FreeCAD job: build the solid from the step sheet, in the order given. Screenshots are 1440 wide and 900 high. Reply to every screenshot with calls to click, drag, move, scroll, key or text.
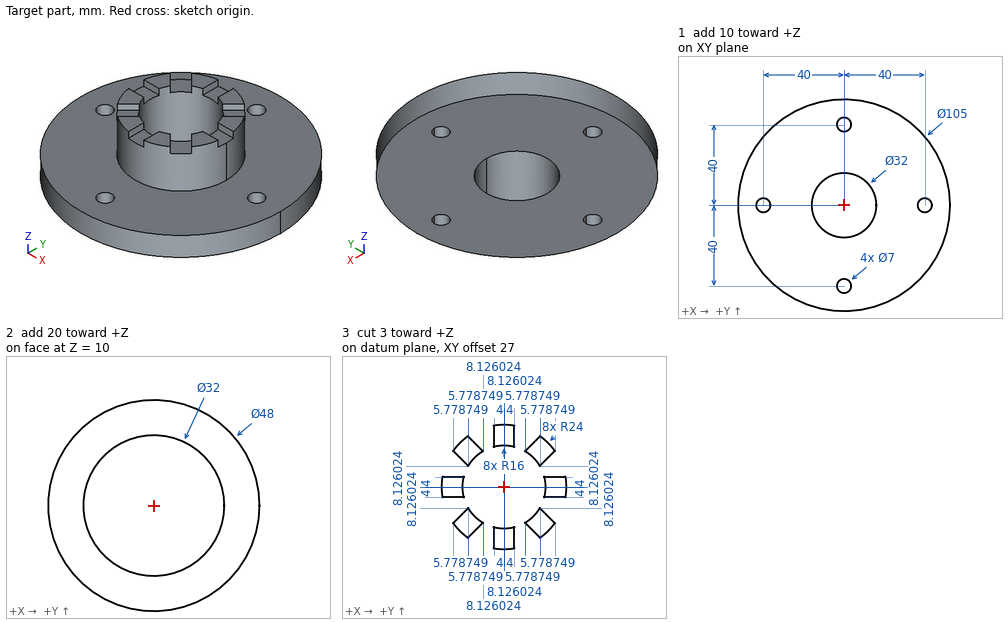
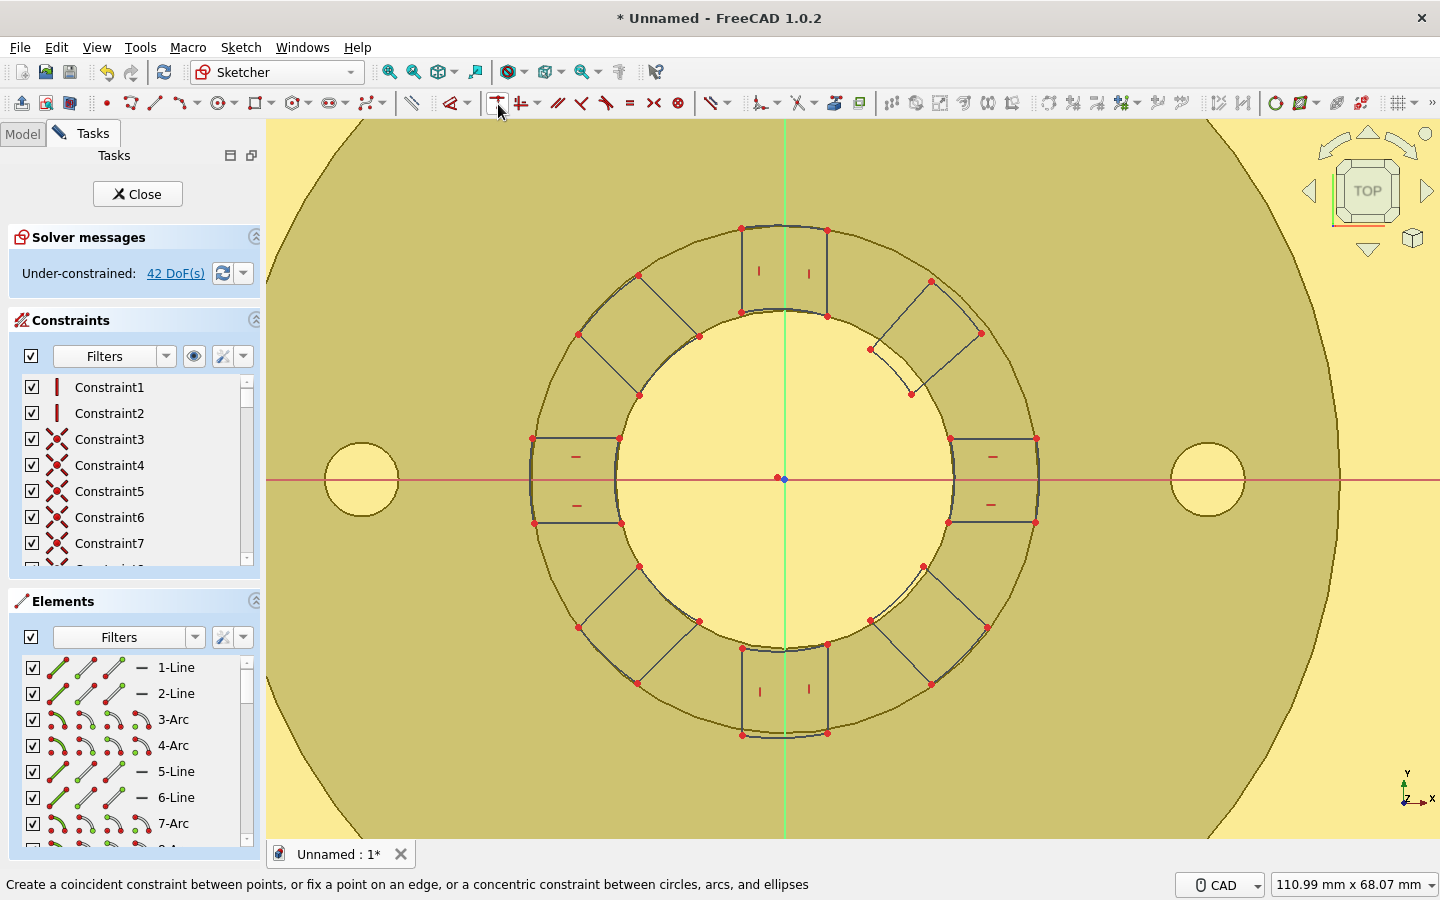
drag(768, 467, 795, 490)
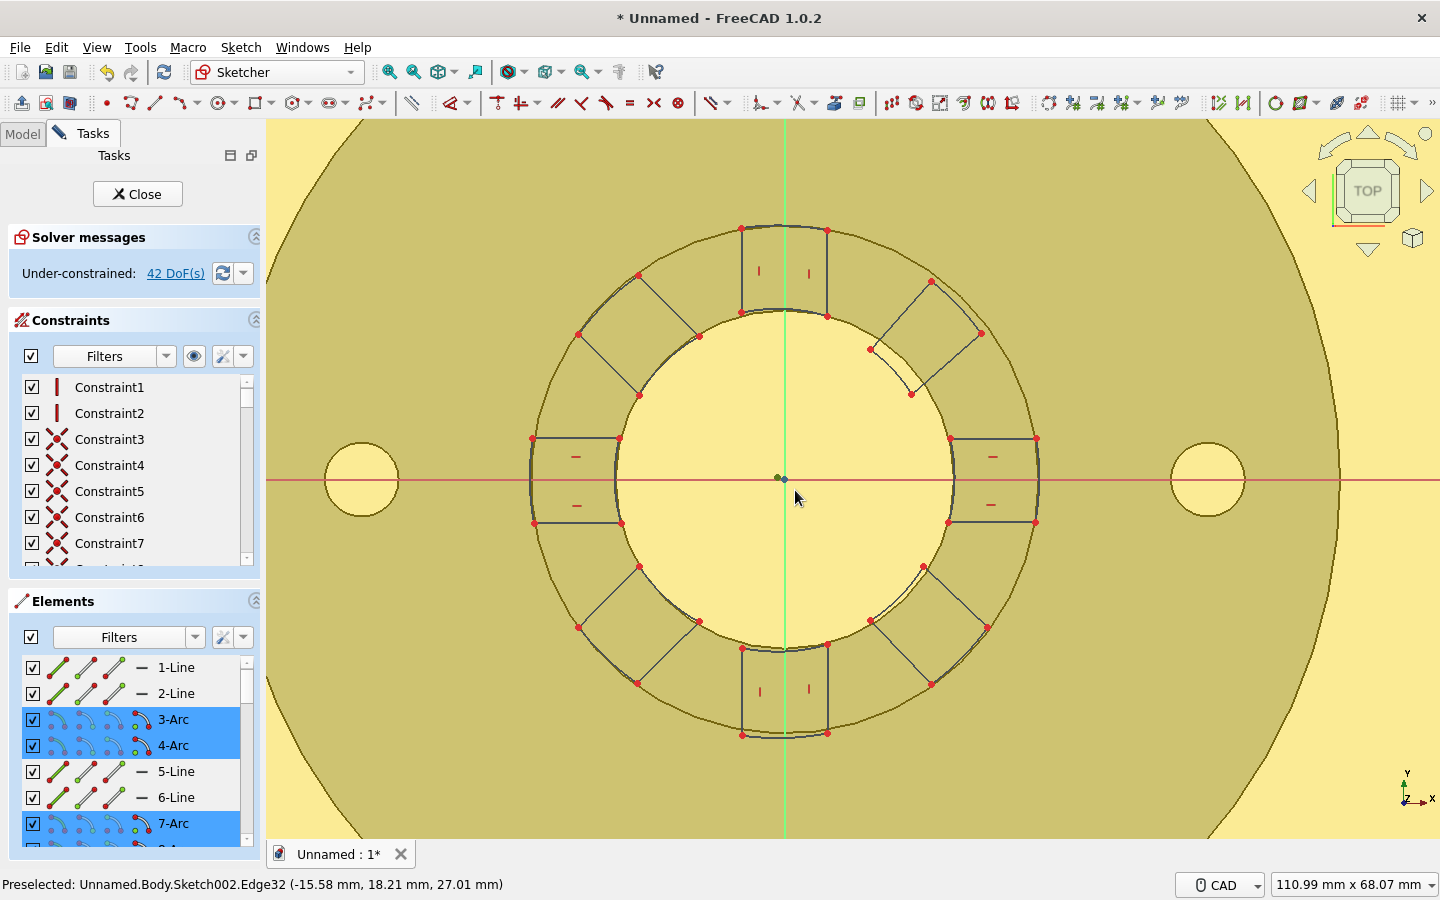
click(498, 104)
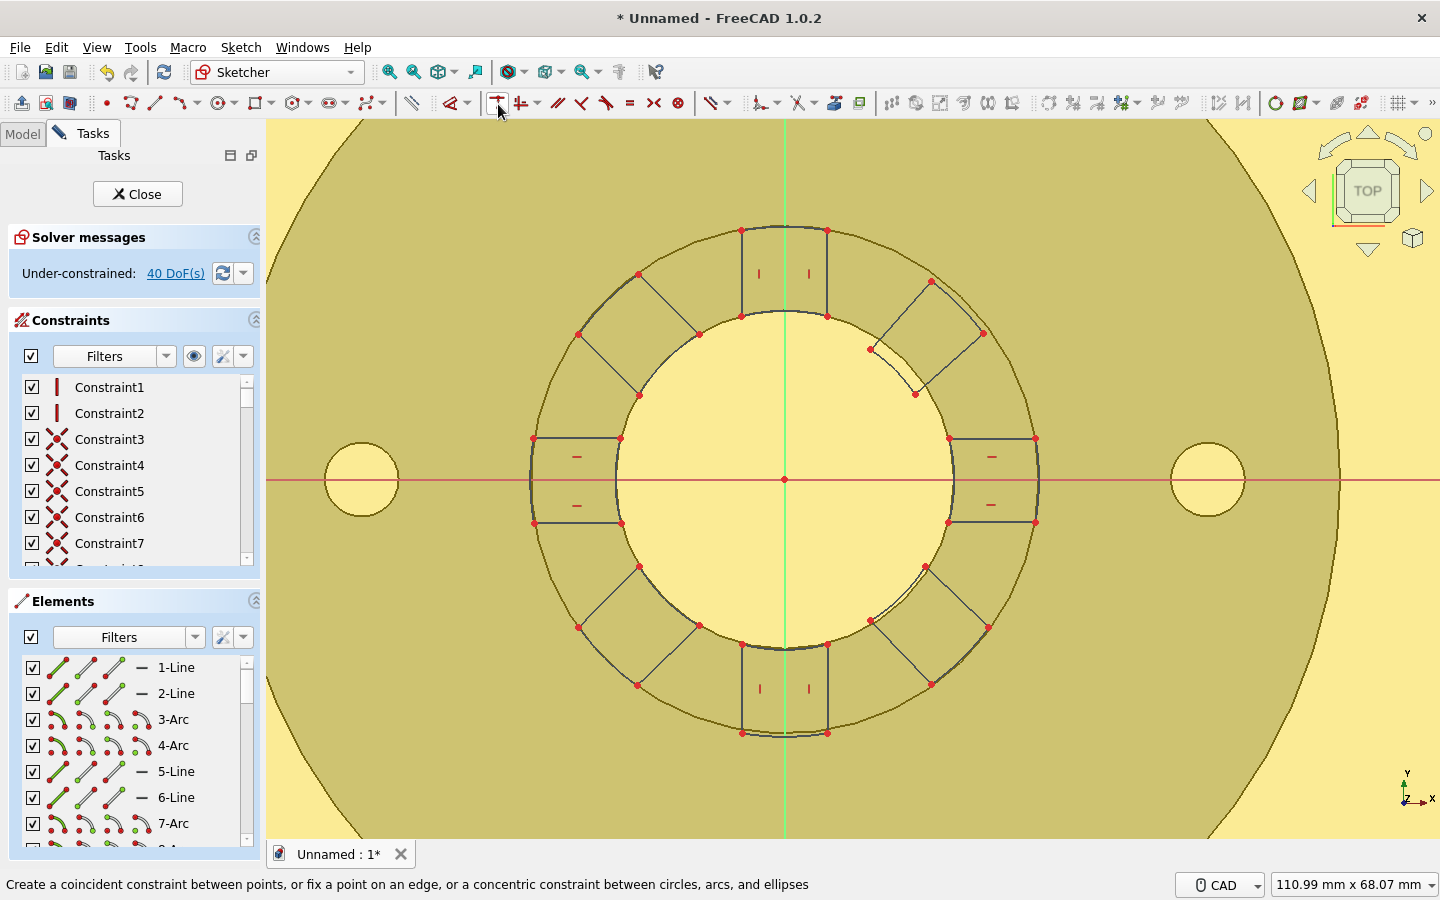
click(802, 312)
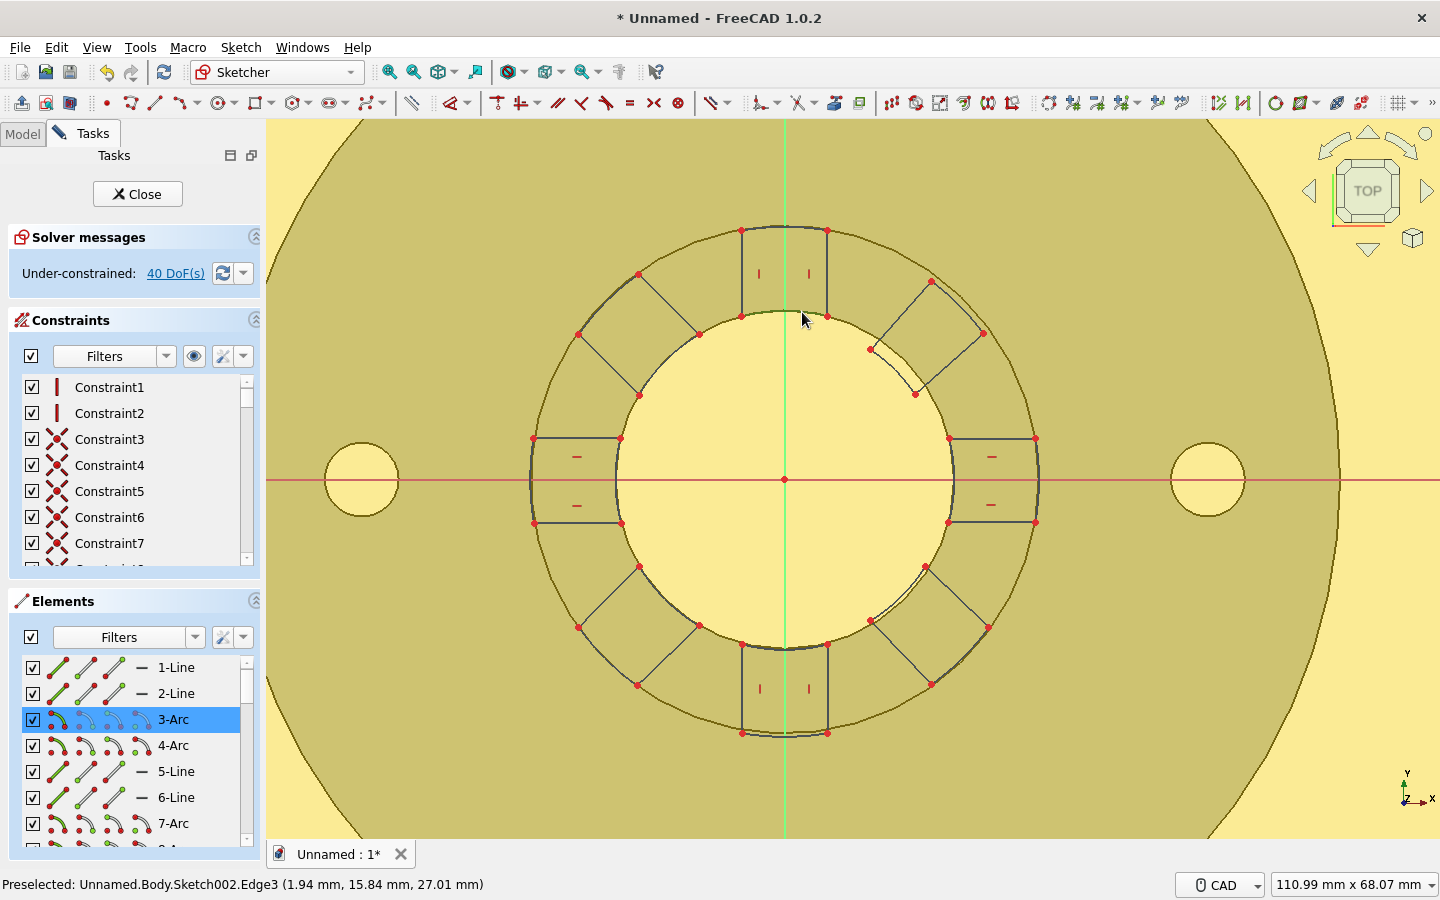
click(904, 379)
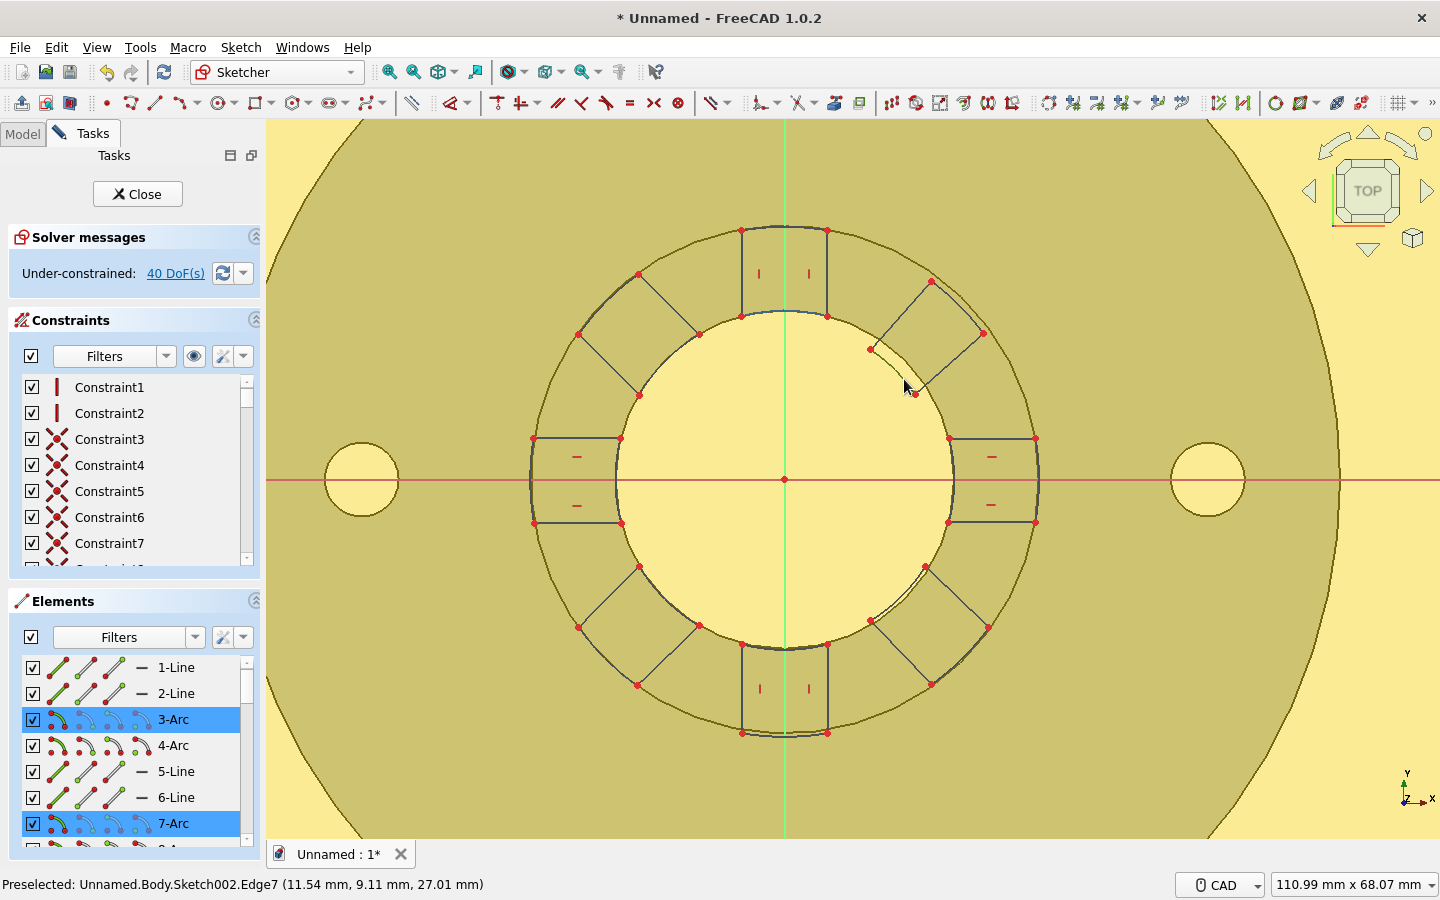
click(953, 497)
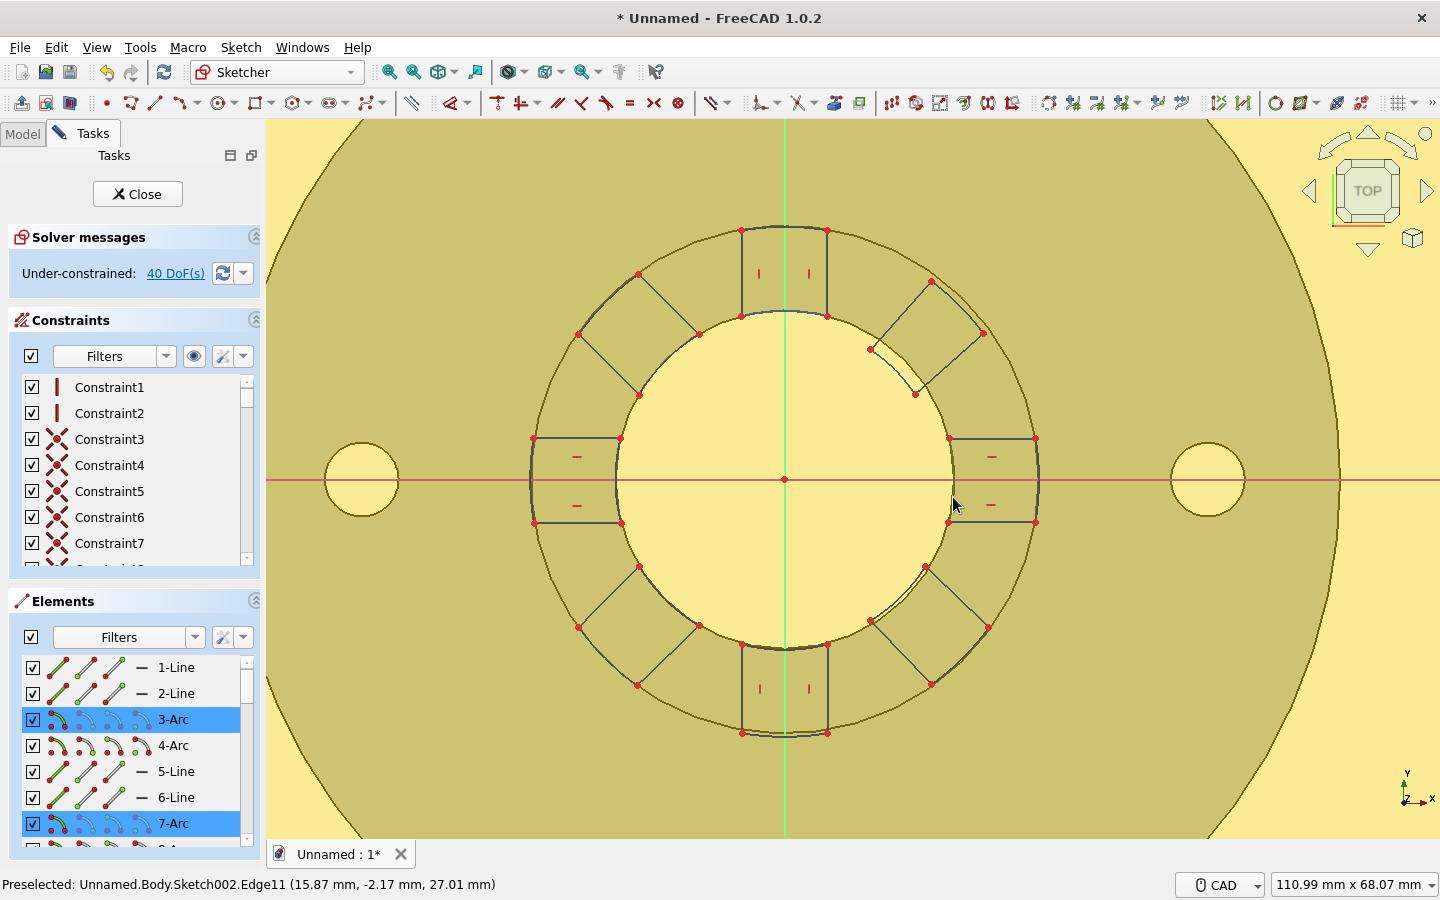
click(890, 607)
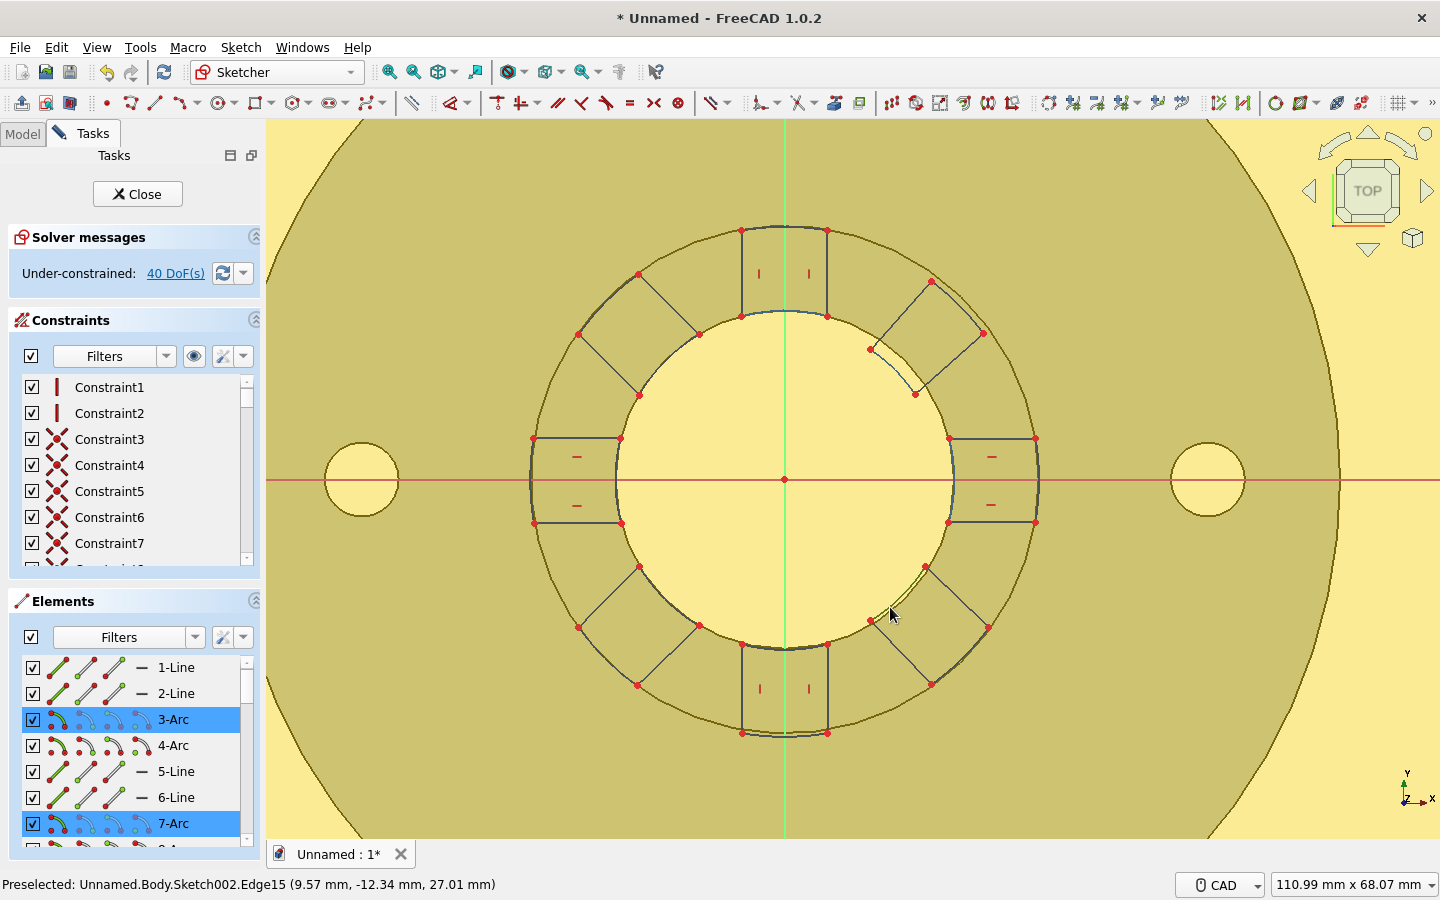
click(768, 649)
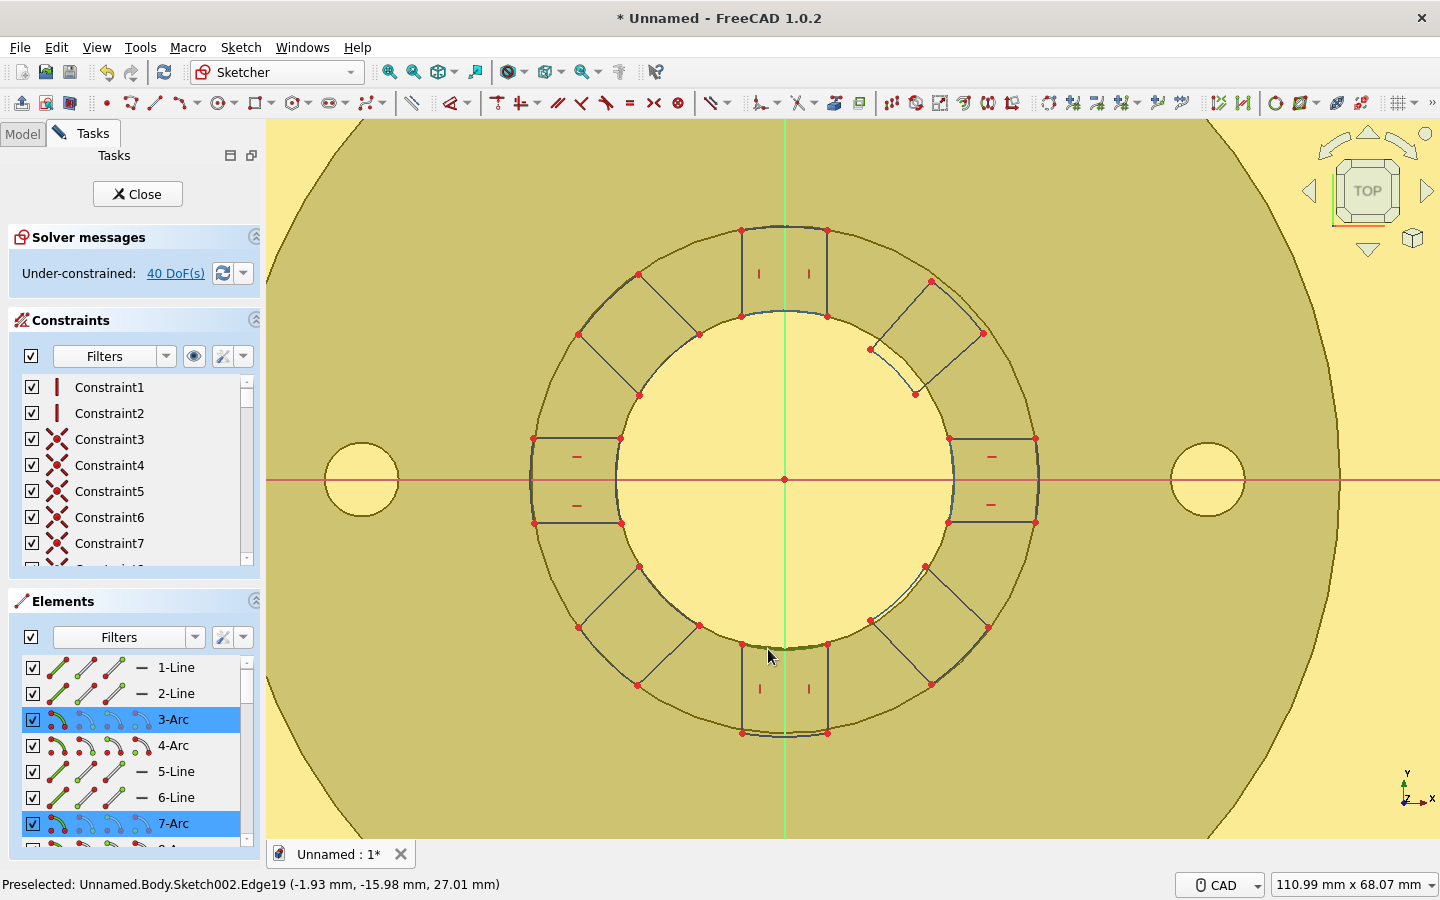
click(654, 587)